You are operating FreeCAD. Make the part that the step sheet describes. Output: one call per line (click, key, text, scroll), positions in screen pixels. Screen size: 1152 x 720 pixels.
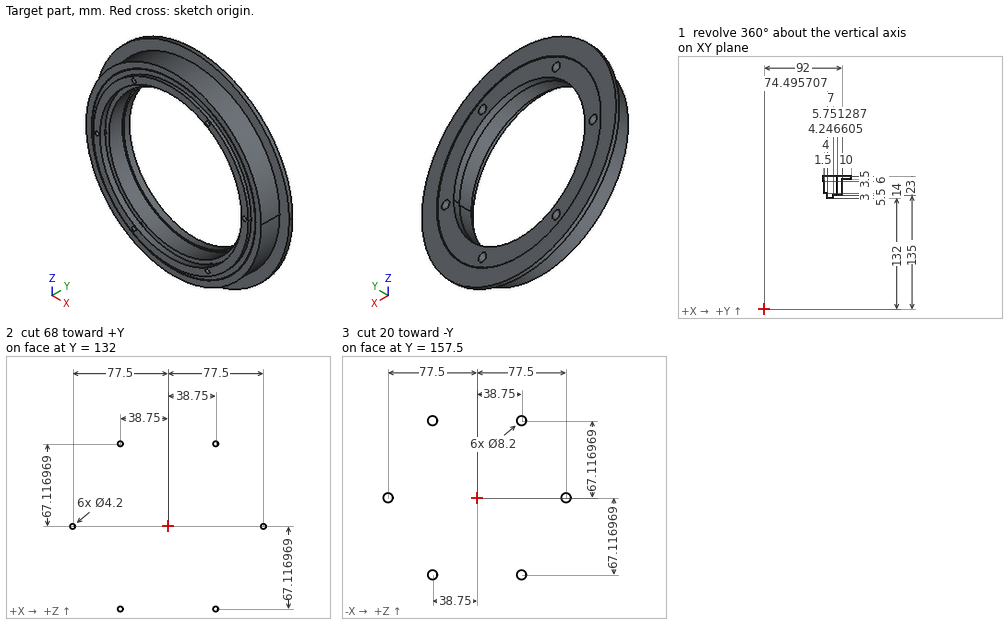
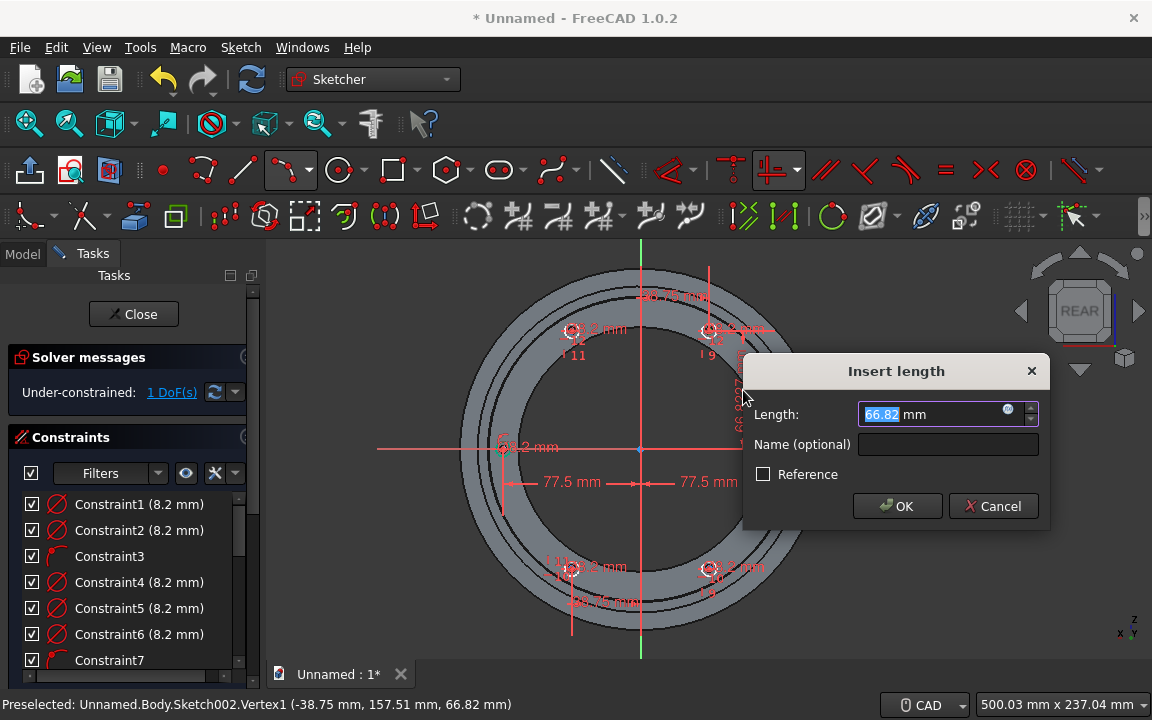
text(67.116969)
key(Return)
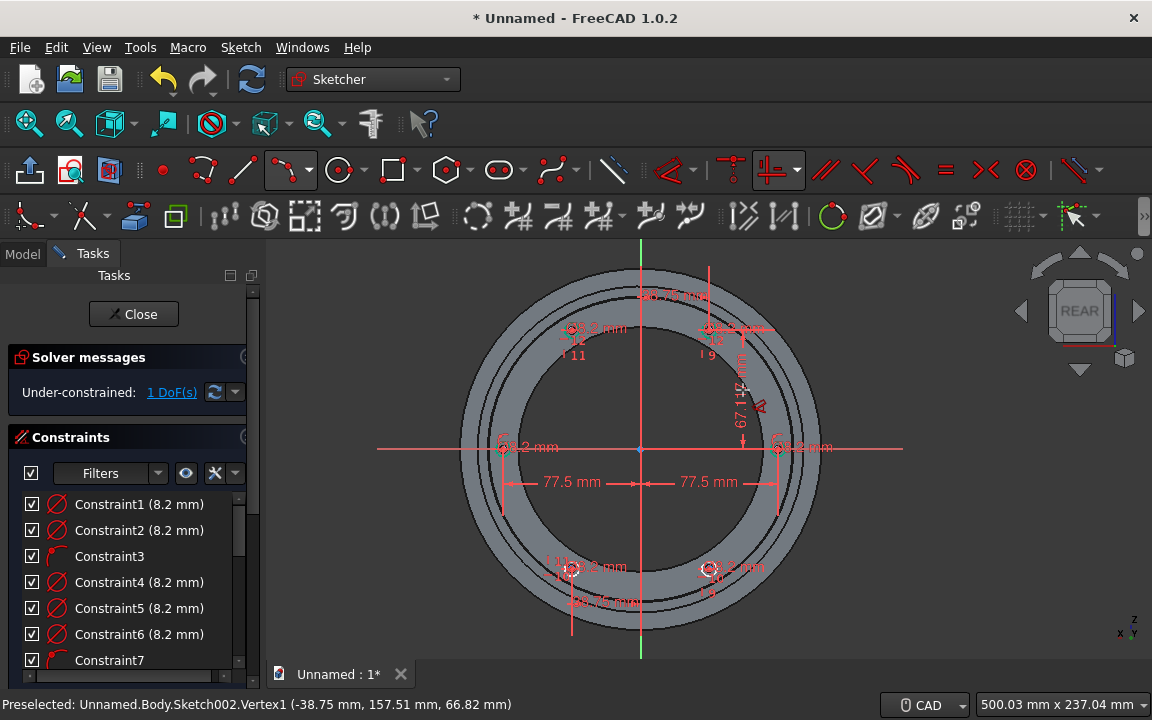
click(709, 569)
click(743, 509)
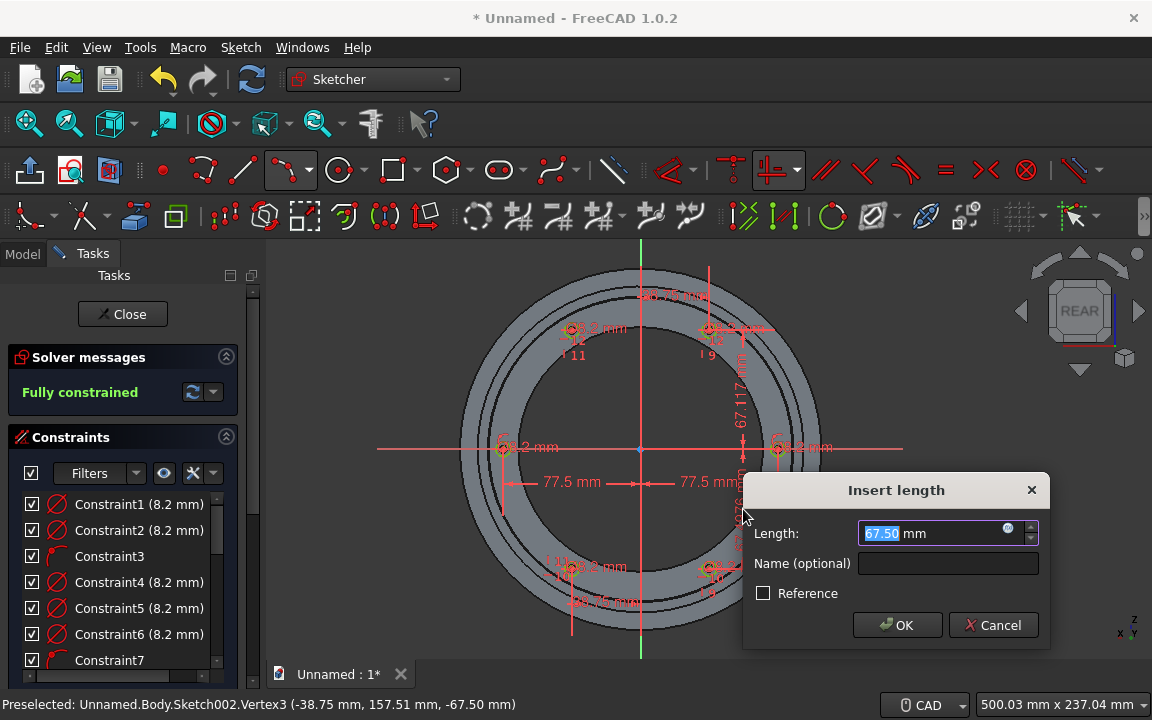
text(67.116969)
key(Return)
key(Escape)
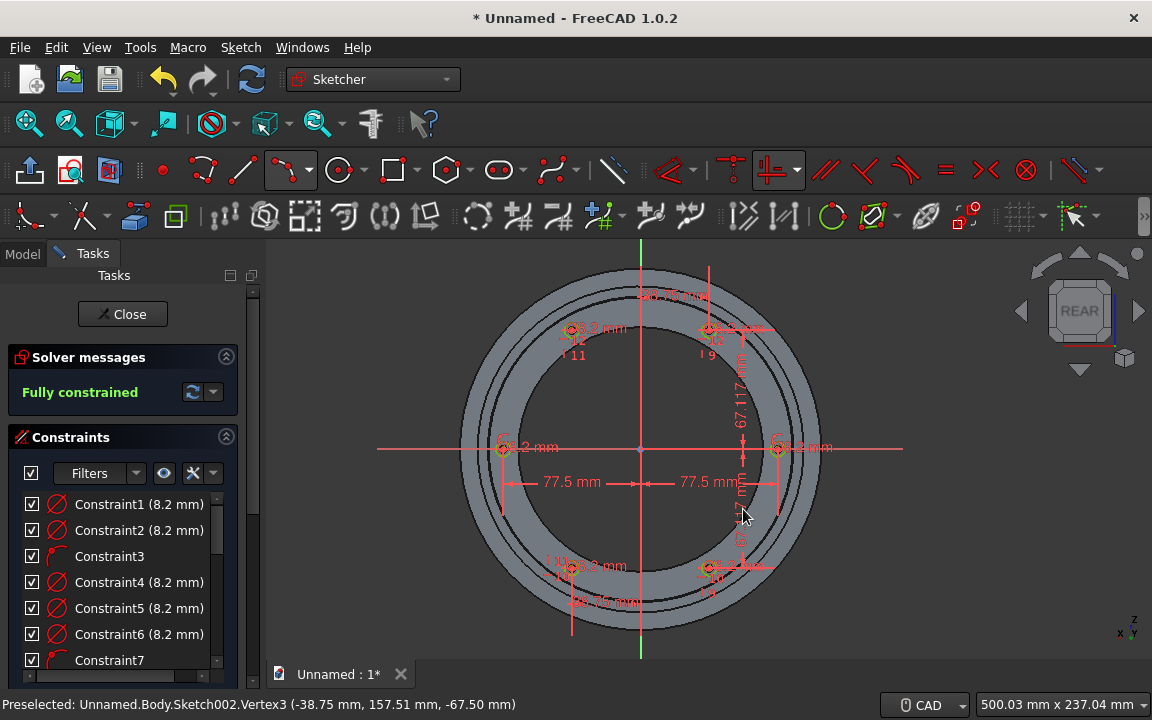
click(123, 314)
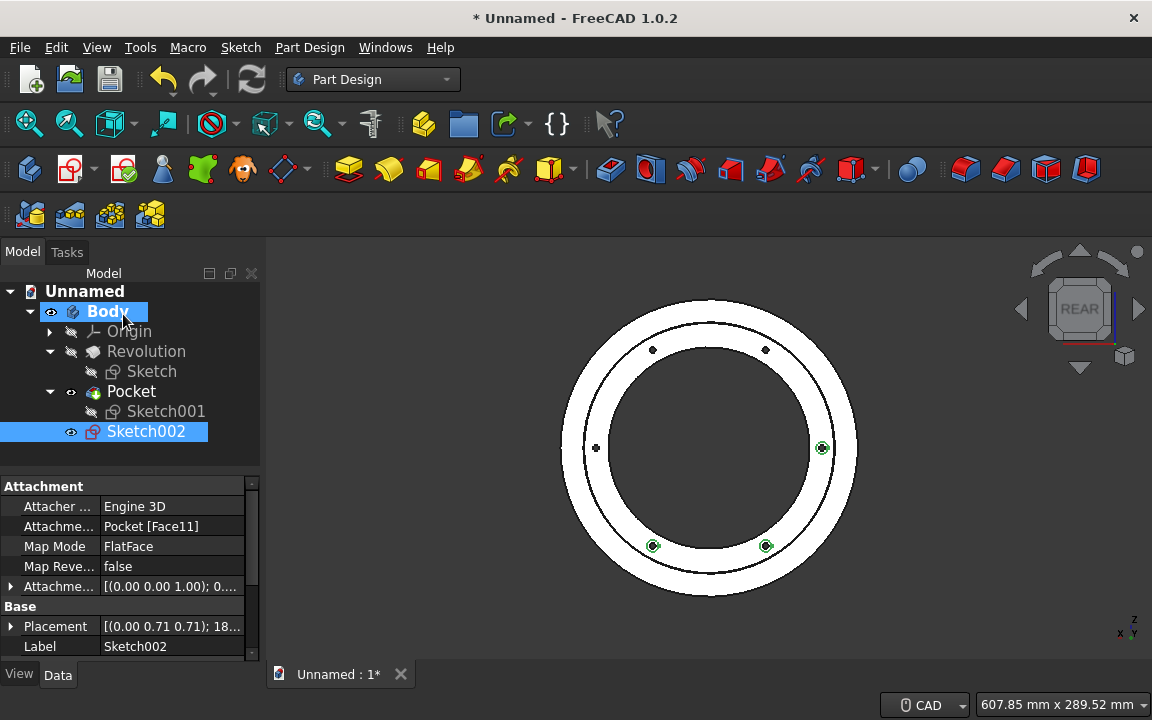
click(612, 170)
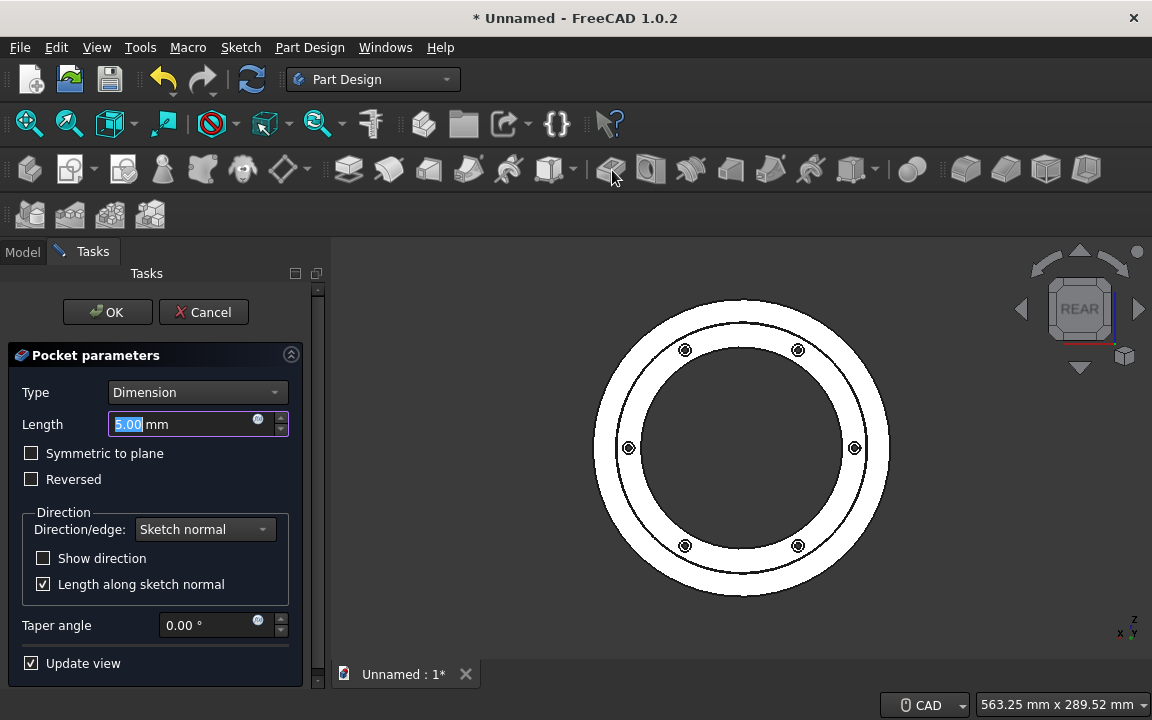
text(20)
key(Tab)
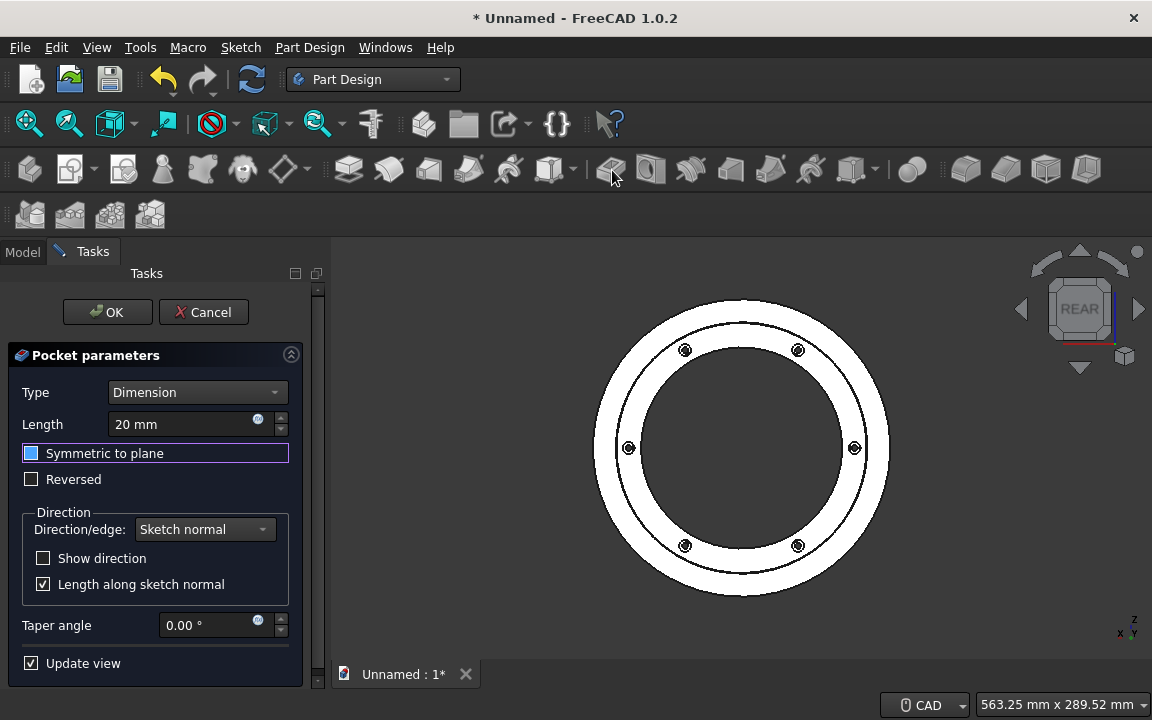
click(108, 312)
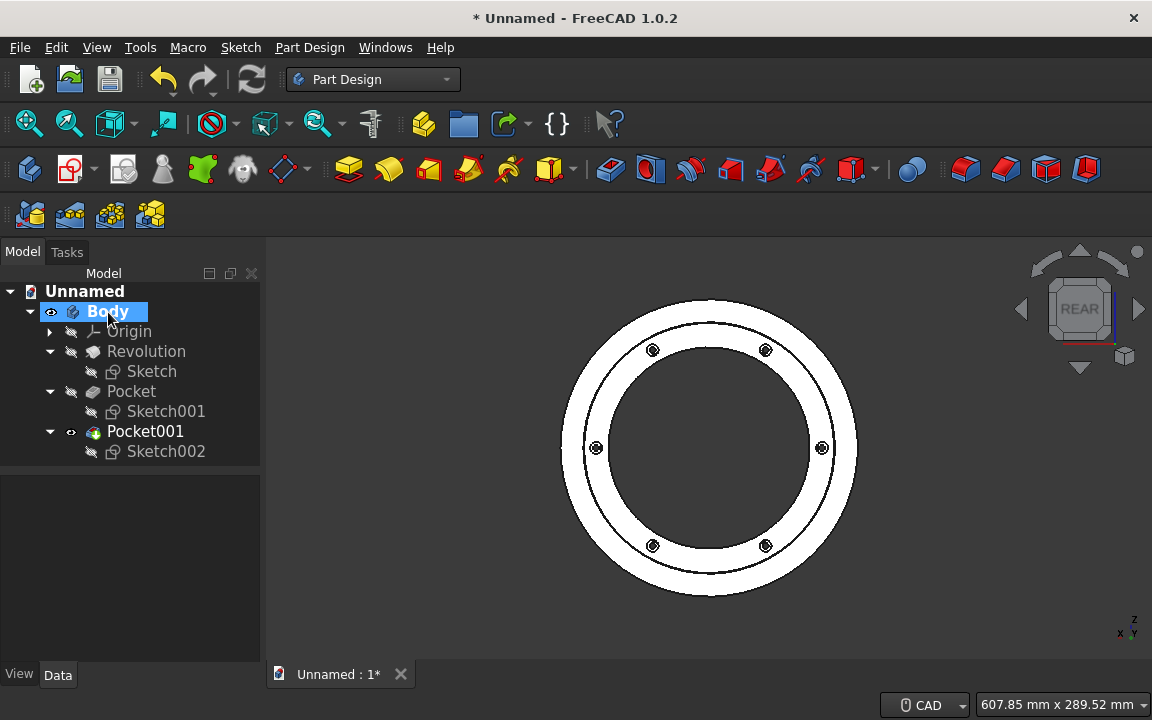
key(0)